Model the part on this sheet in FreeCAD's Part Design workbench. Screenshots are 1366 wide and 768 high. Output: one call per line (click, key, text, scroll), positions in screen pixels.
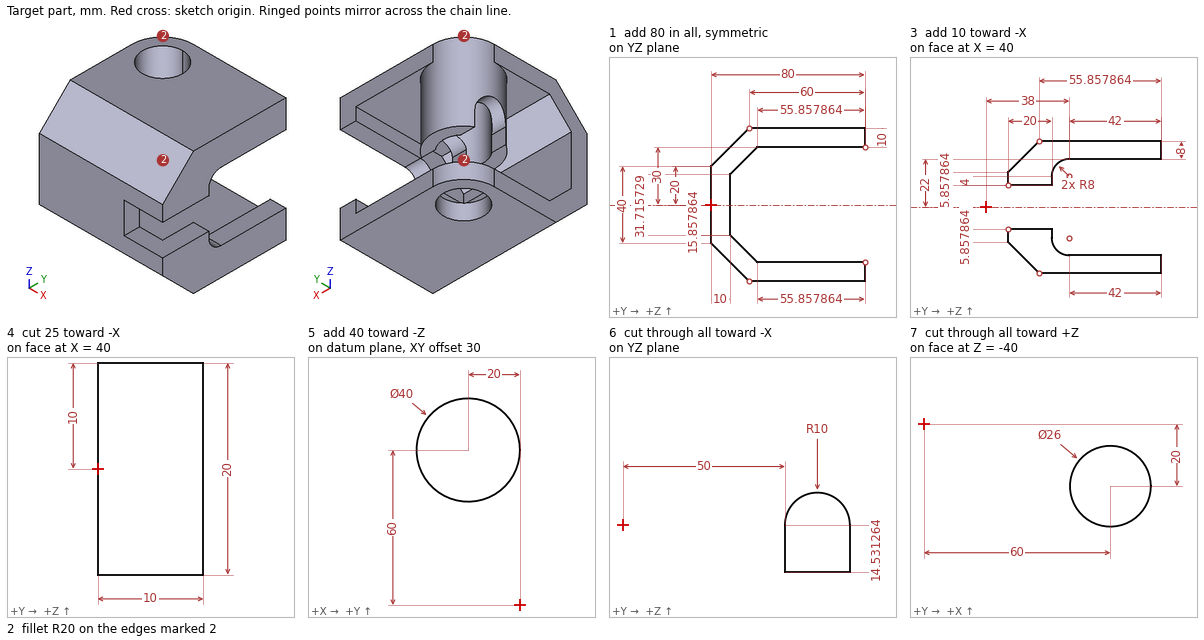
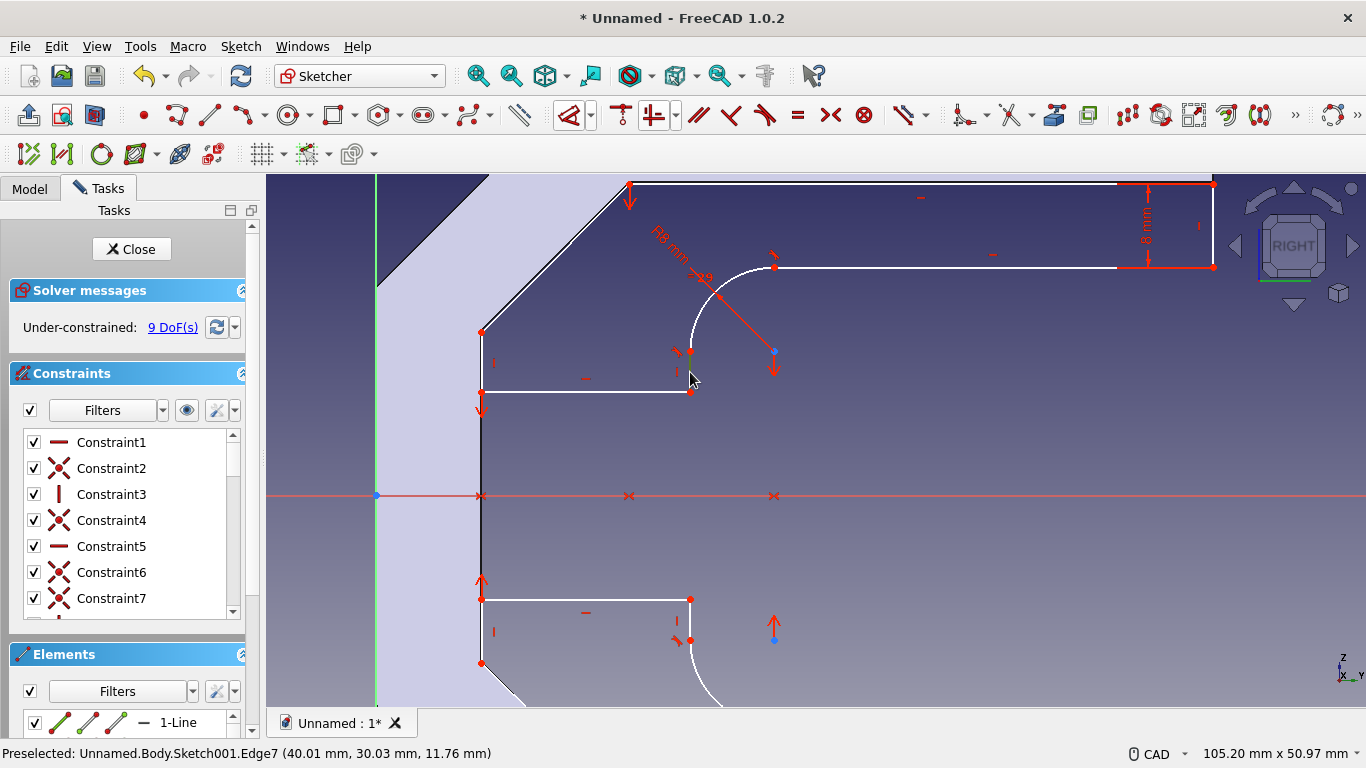
key(i)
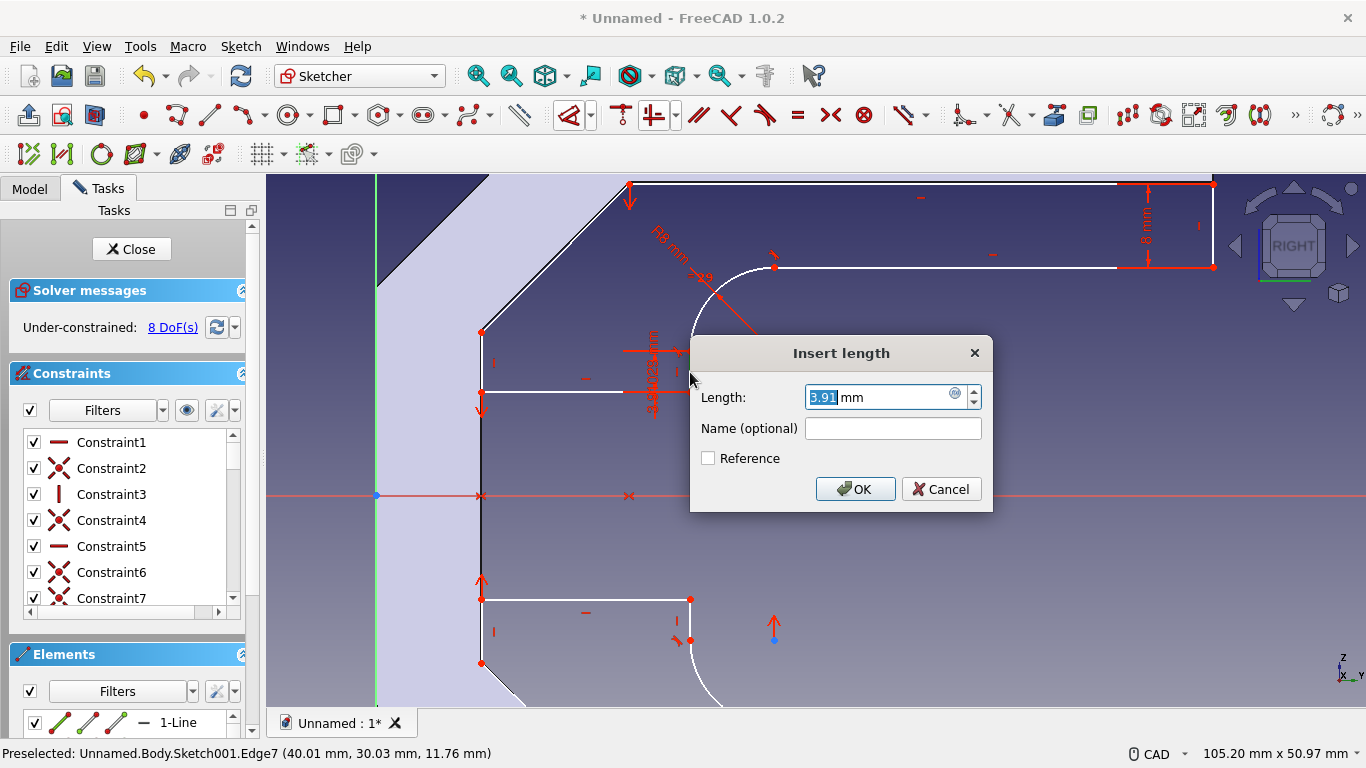
text(4)
key(Return)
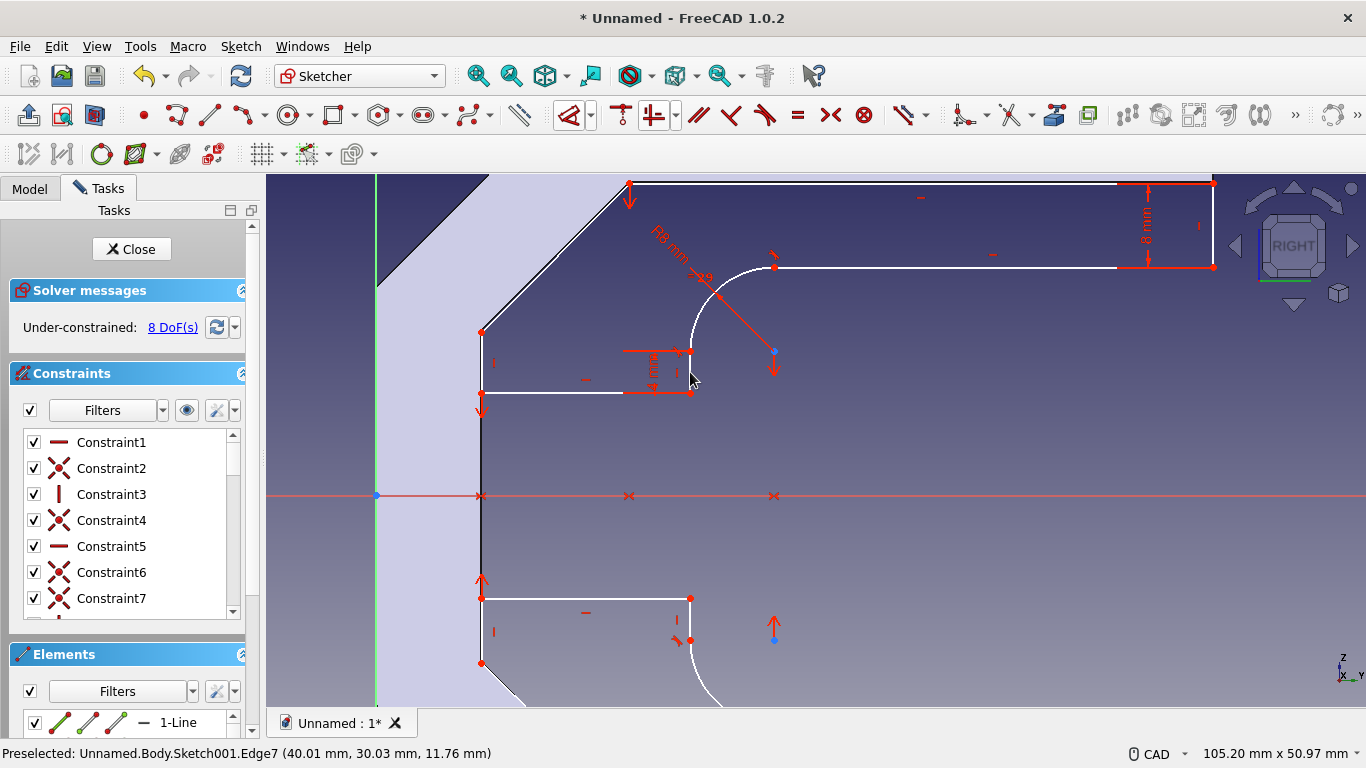
click(906, 268)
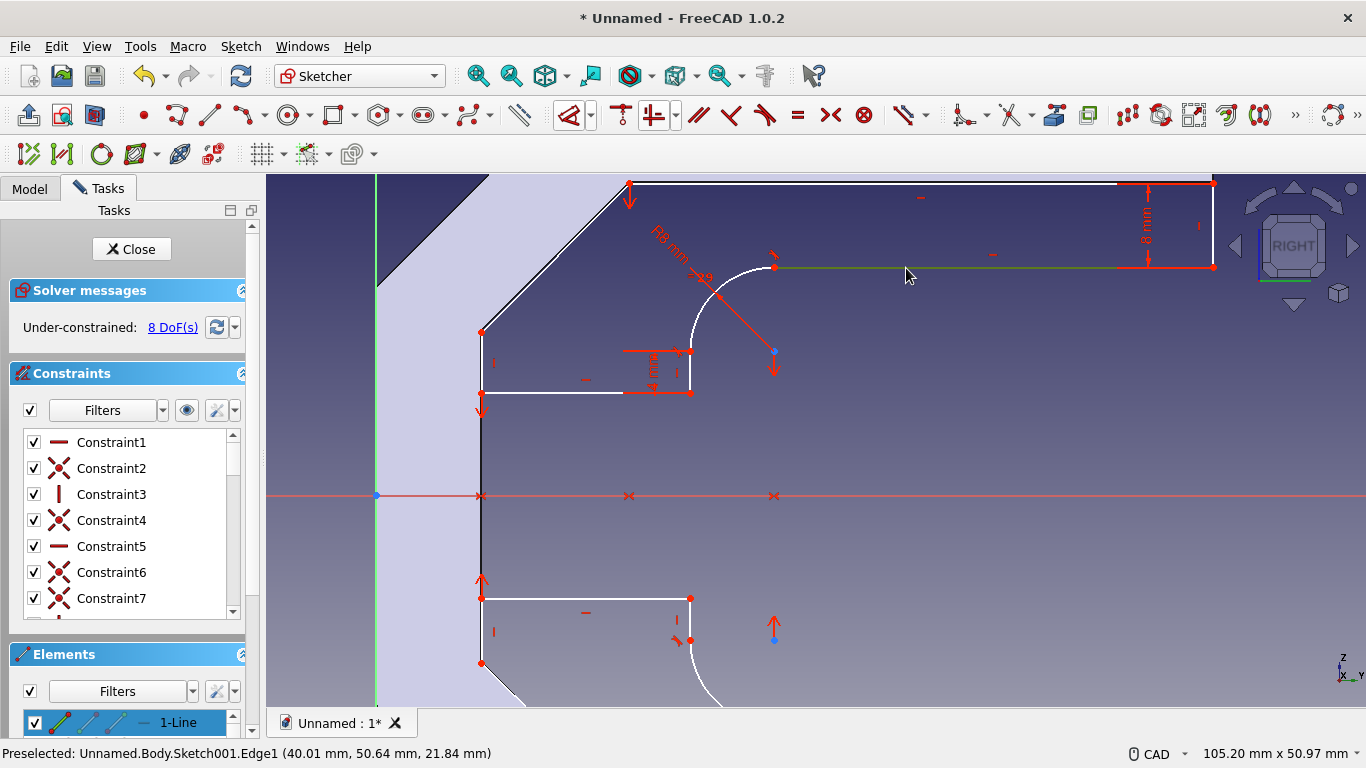
key(l)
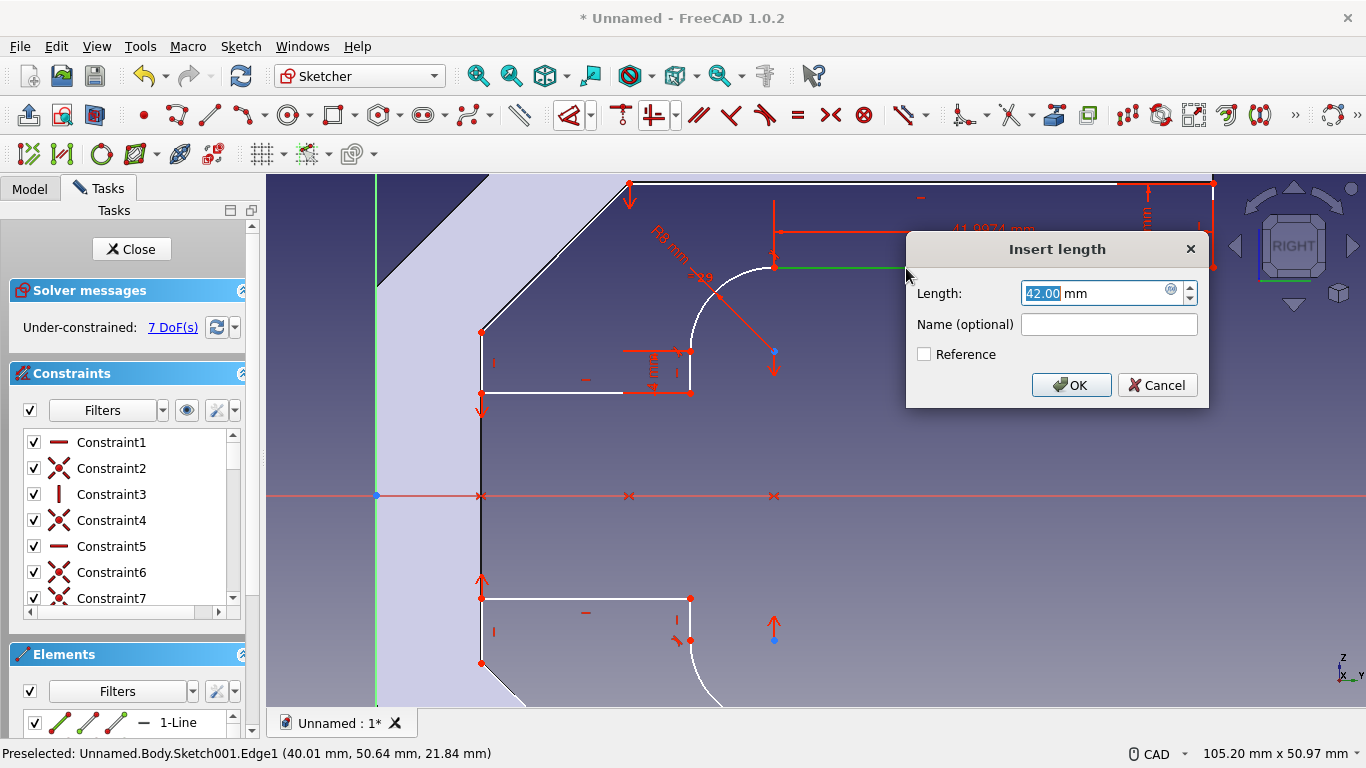
text(42)
key(Return)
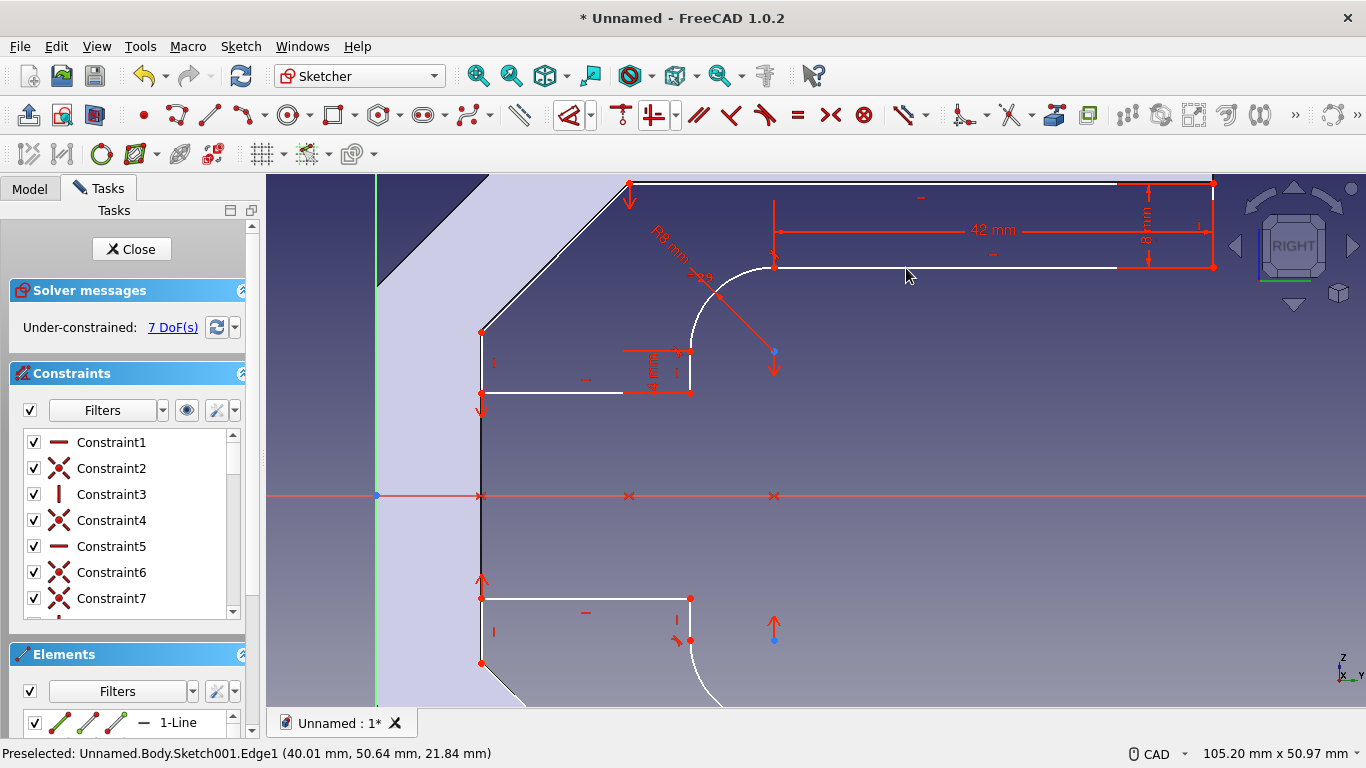
click(544, 393)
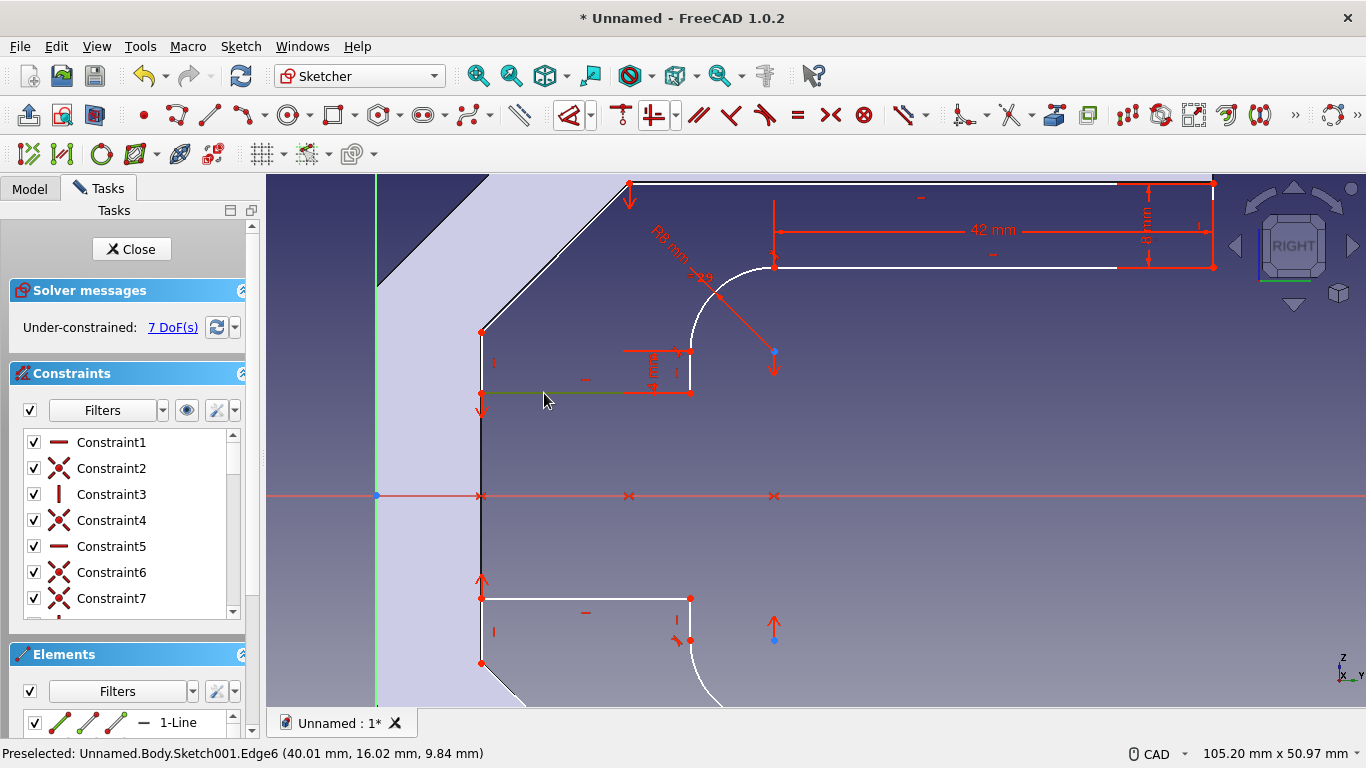
click(590, 116)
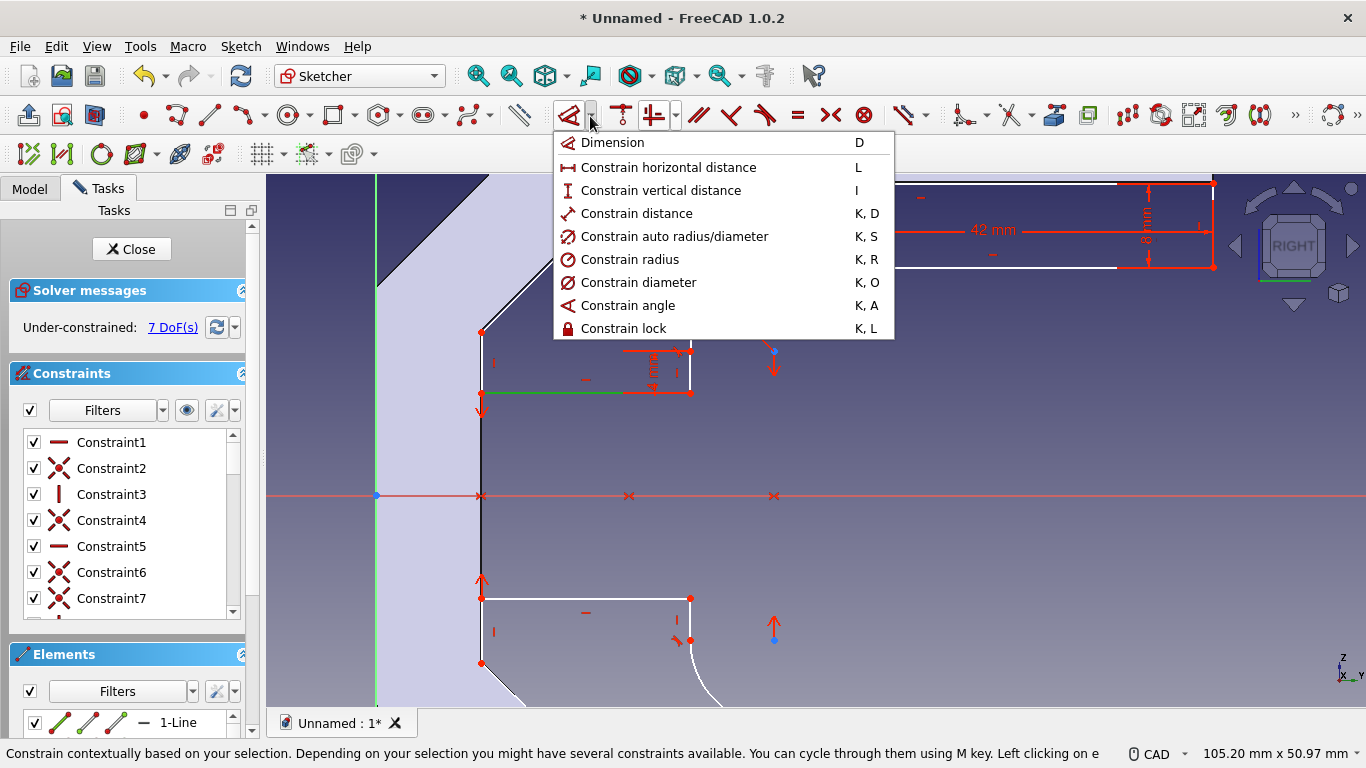
click(724, 168)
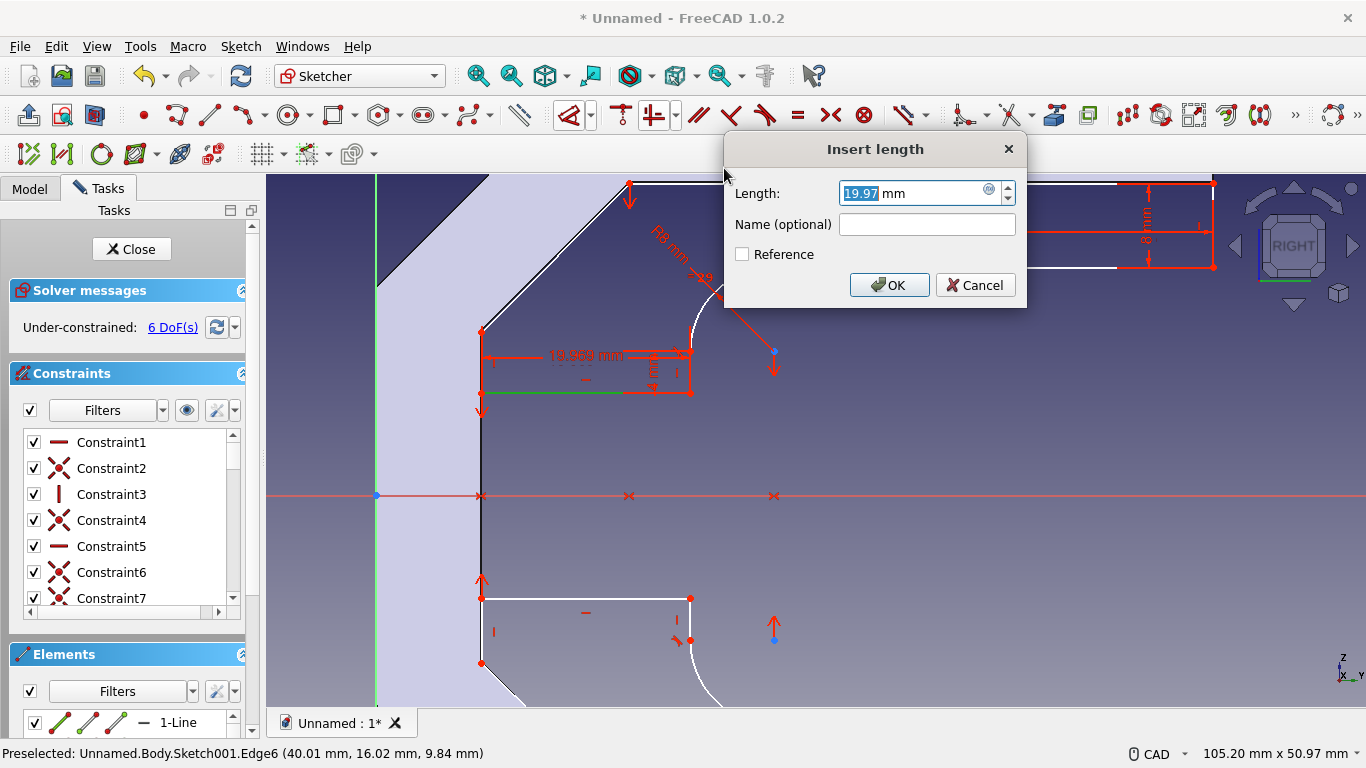
text(20)
key(Return)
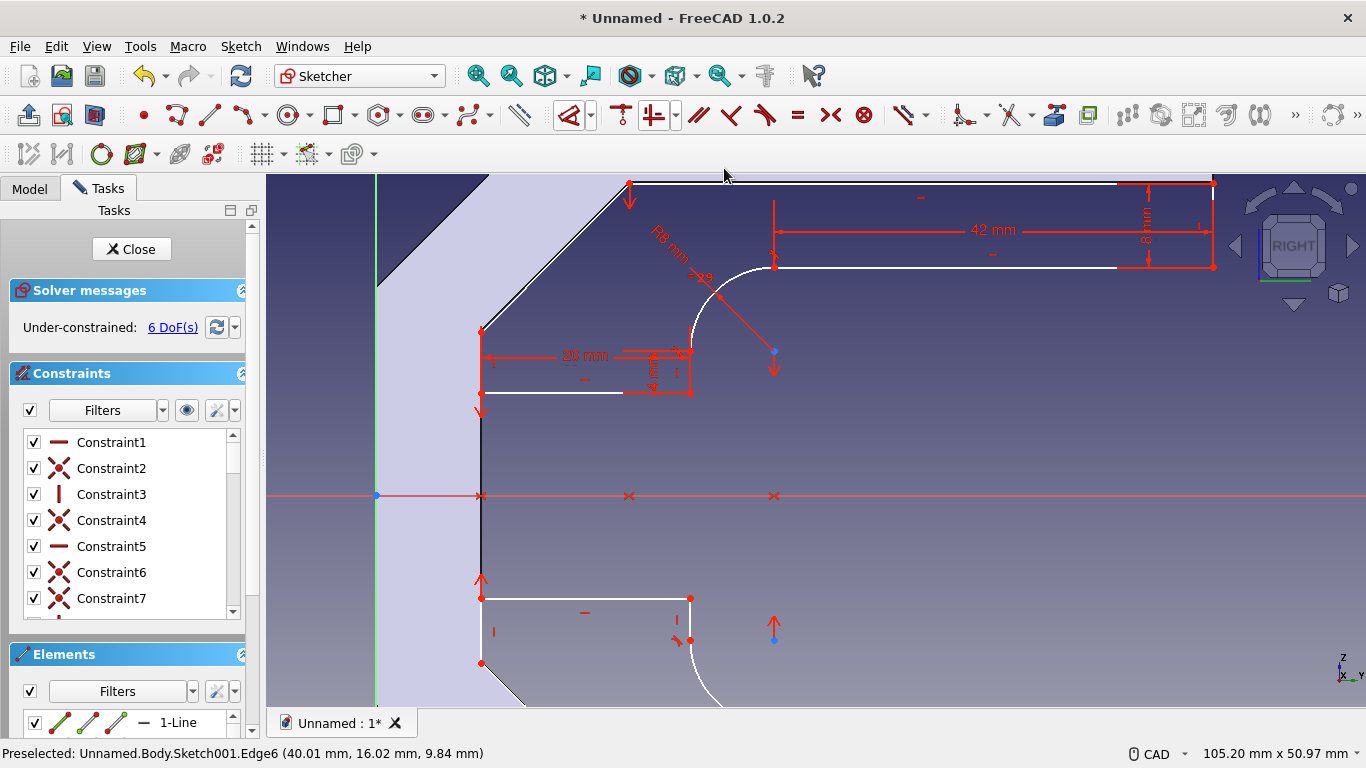
scroll(690, 373, down, 3)